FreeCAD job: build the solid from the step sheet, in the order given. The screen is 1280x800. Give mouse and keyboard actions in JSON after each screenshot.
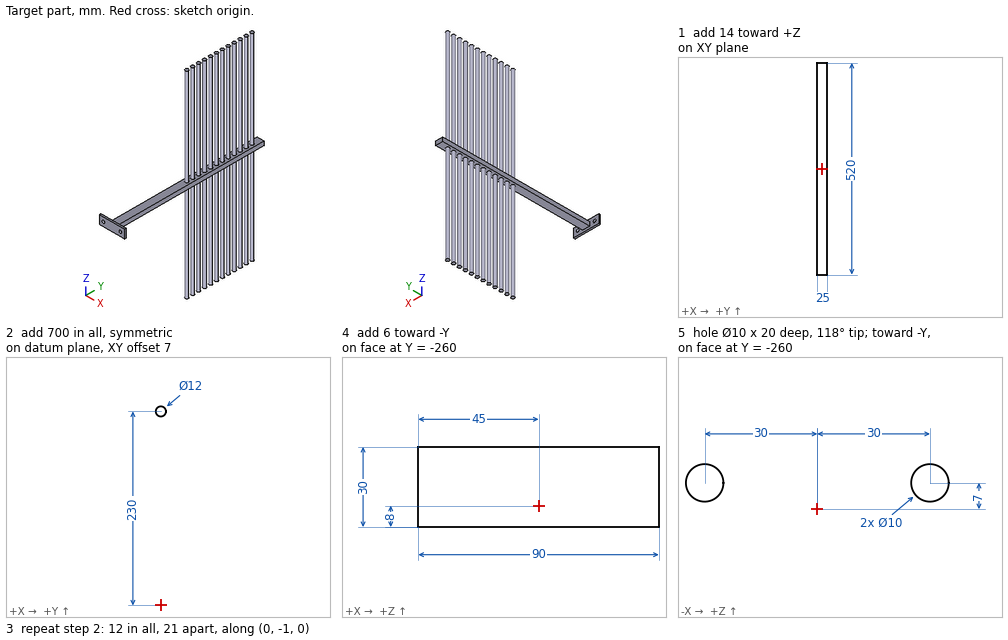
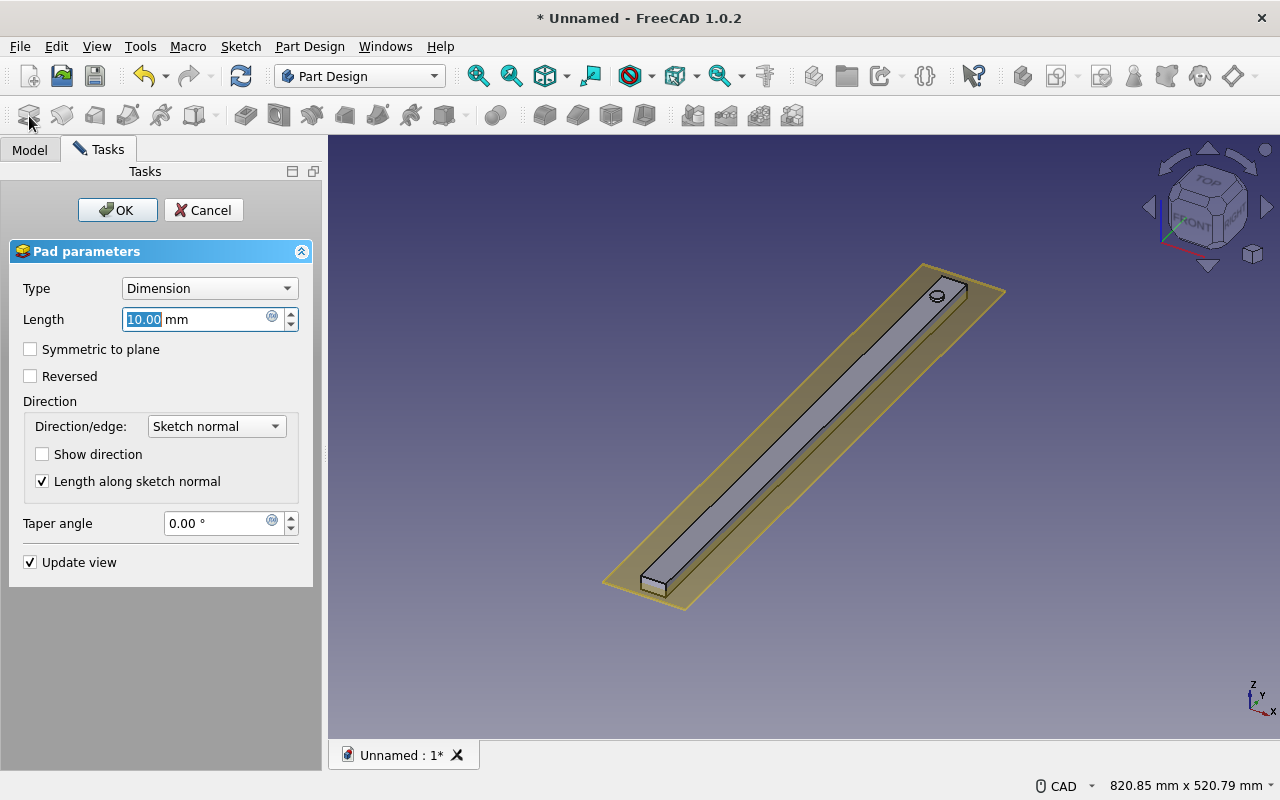
{"action": "type", "text": "700"}
{"action": "key", "text": "Tab"}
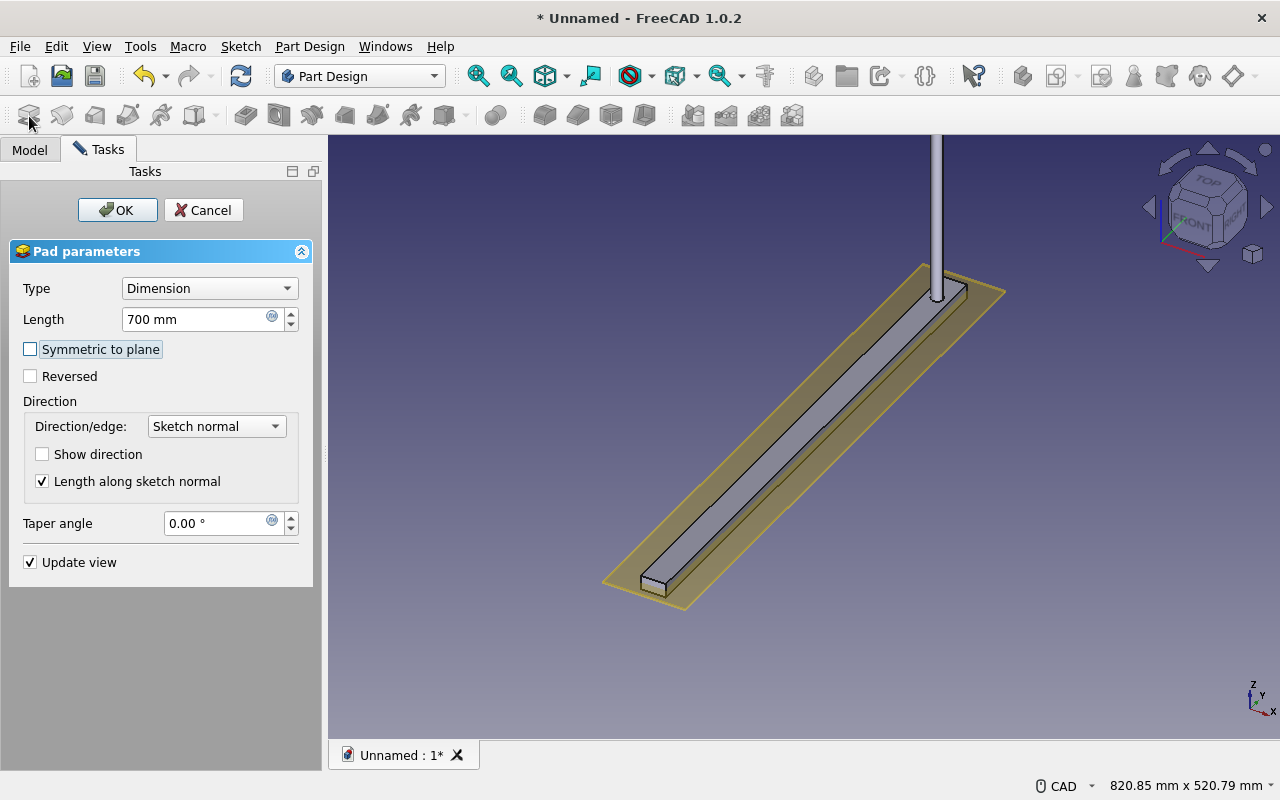
{"action": "left_click", "coordinate": [31, 349]}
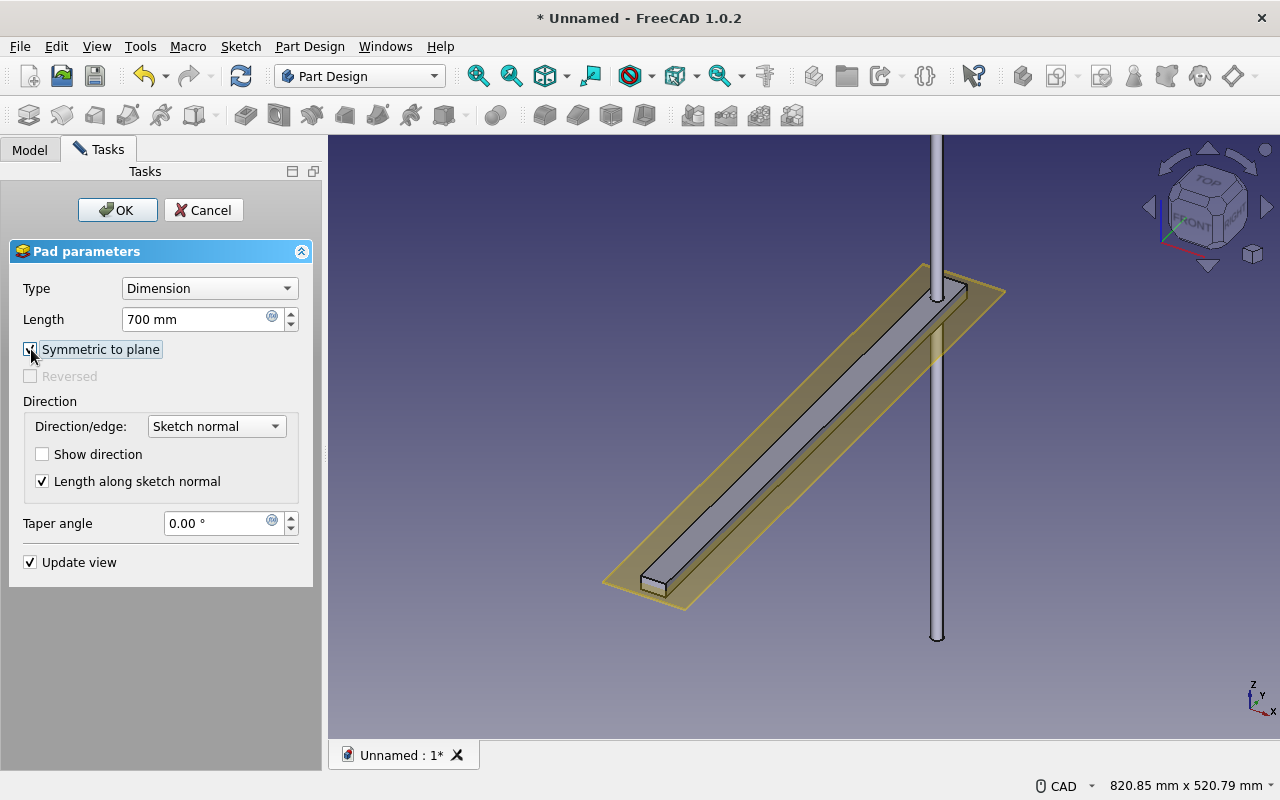
{"action": "left_click", "coordinate": [118, 210]}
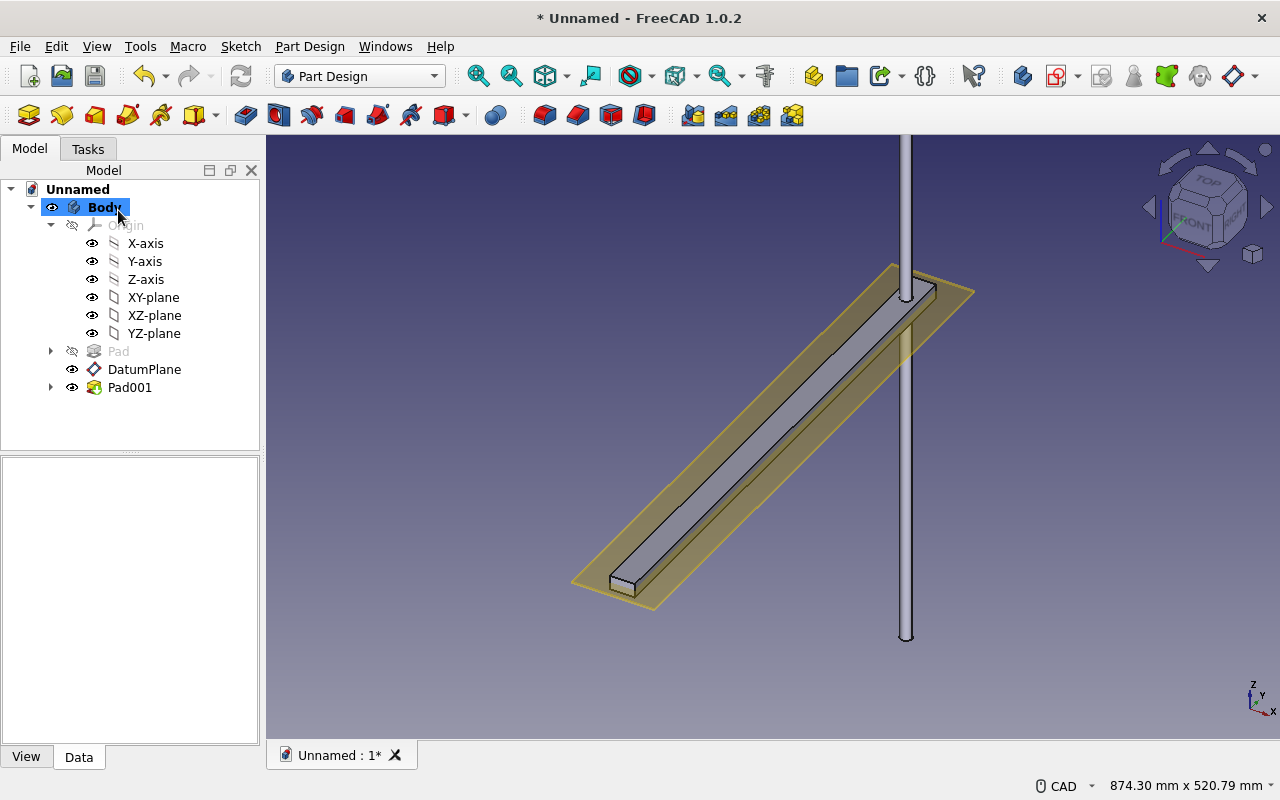
{"action": "left_click", "coordinate": [117, 369]}
{"action": "key", "text": "space"}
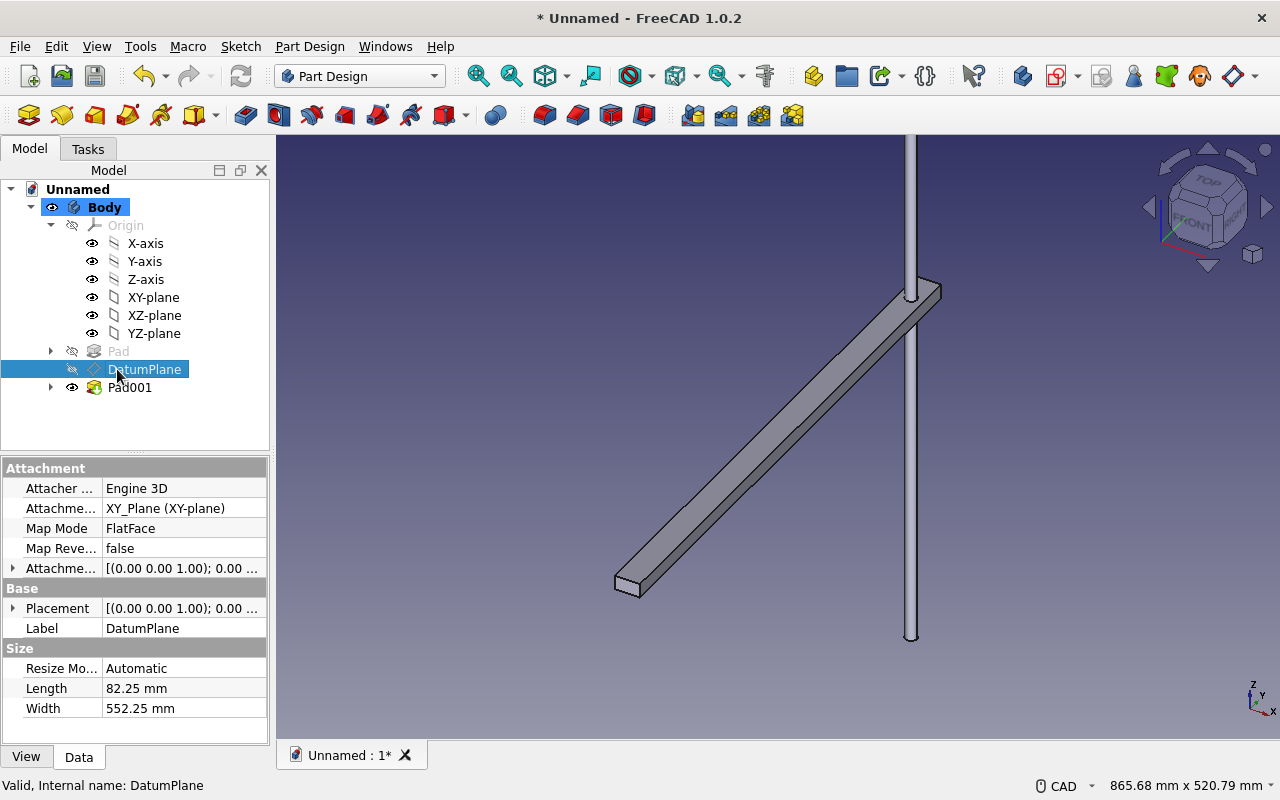
{"action": "left_click", "coordinate": [479, 76]}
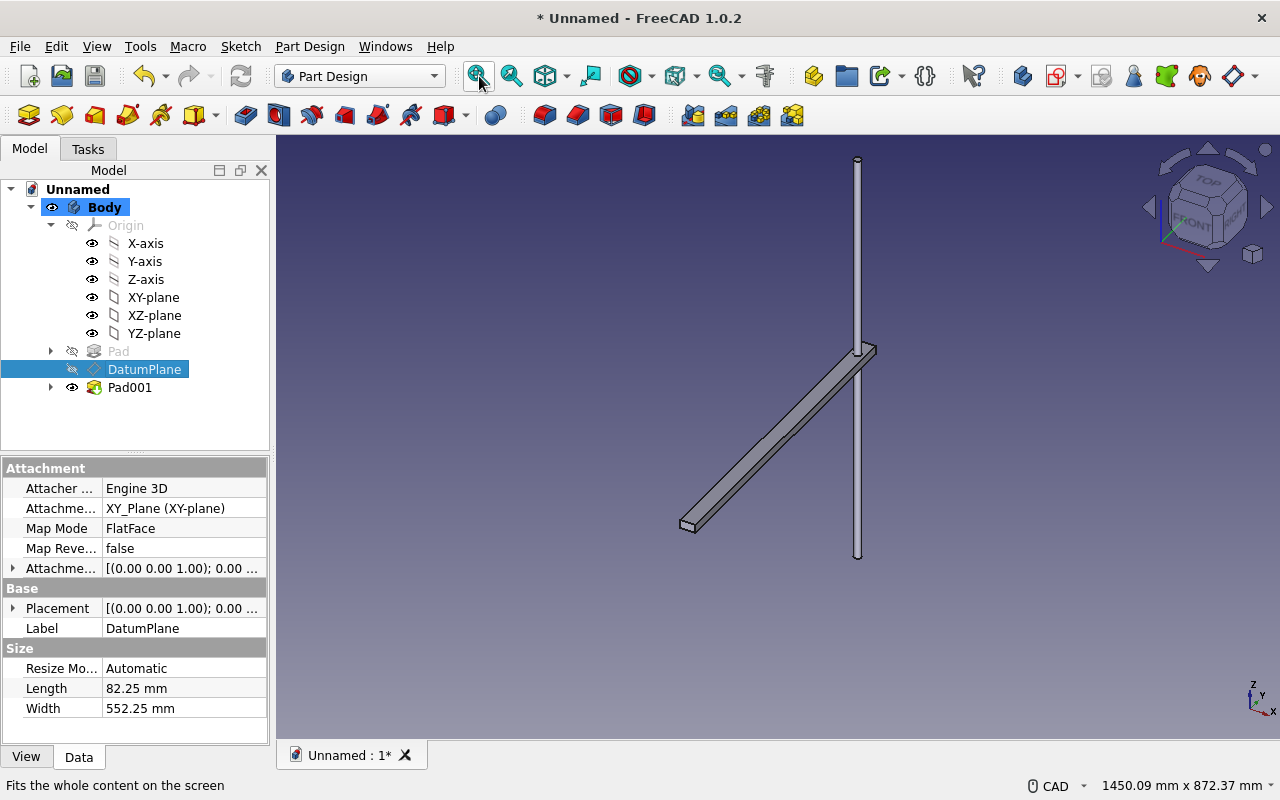
{"action": "left_click", "coordinate": [117, 387]}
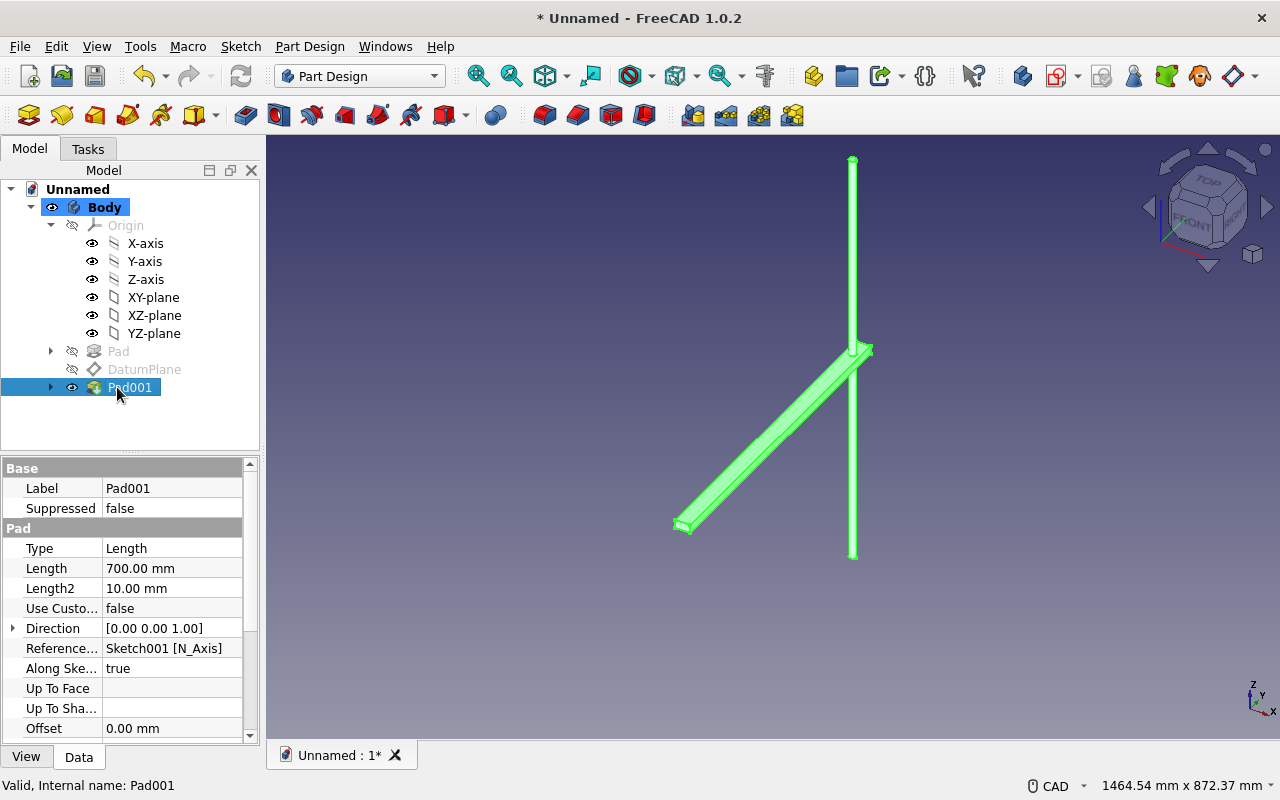
{"action": "left_click", "coordinate": [726, 116]}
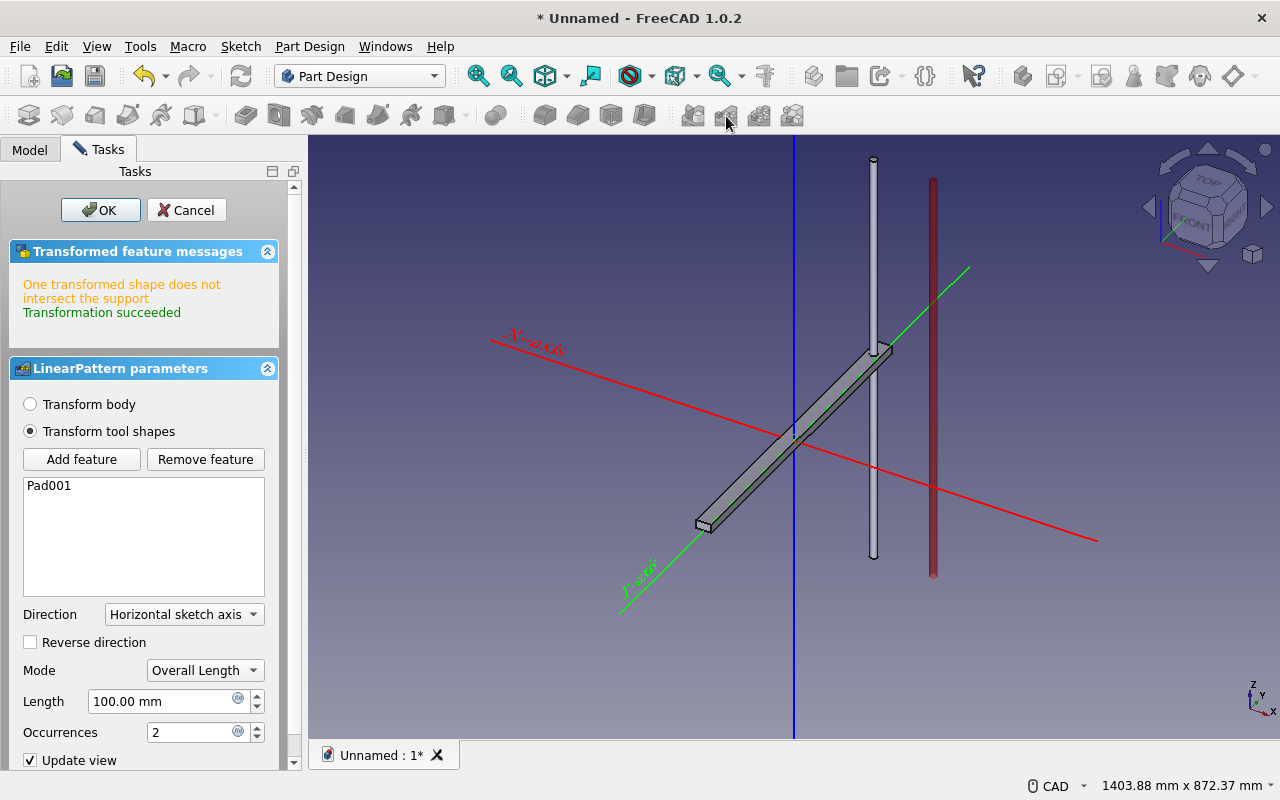
{"action": "left_click", "coordinate": [185, 614]}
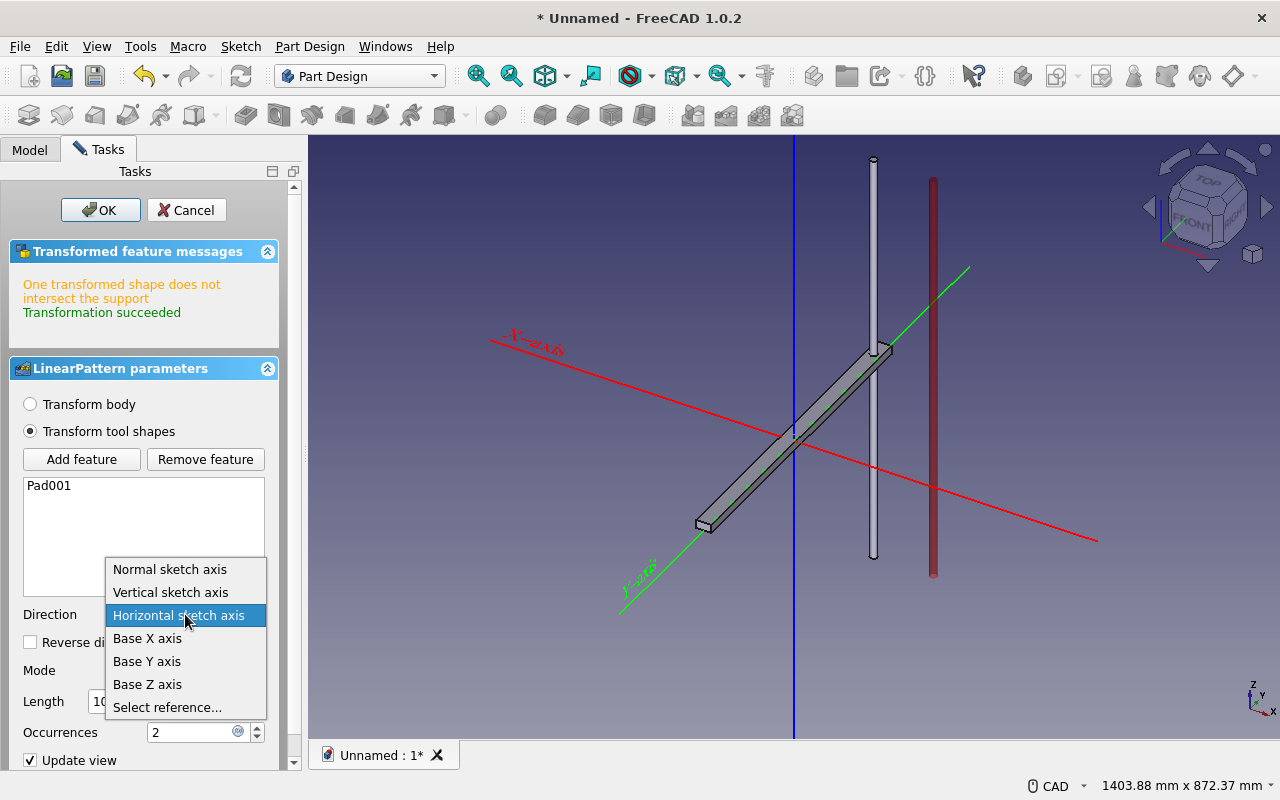
{"action": "left_click", "coordinate": [184, 662]}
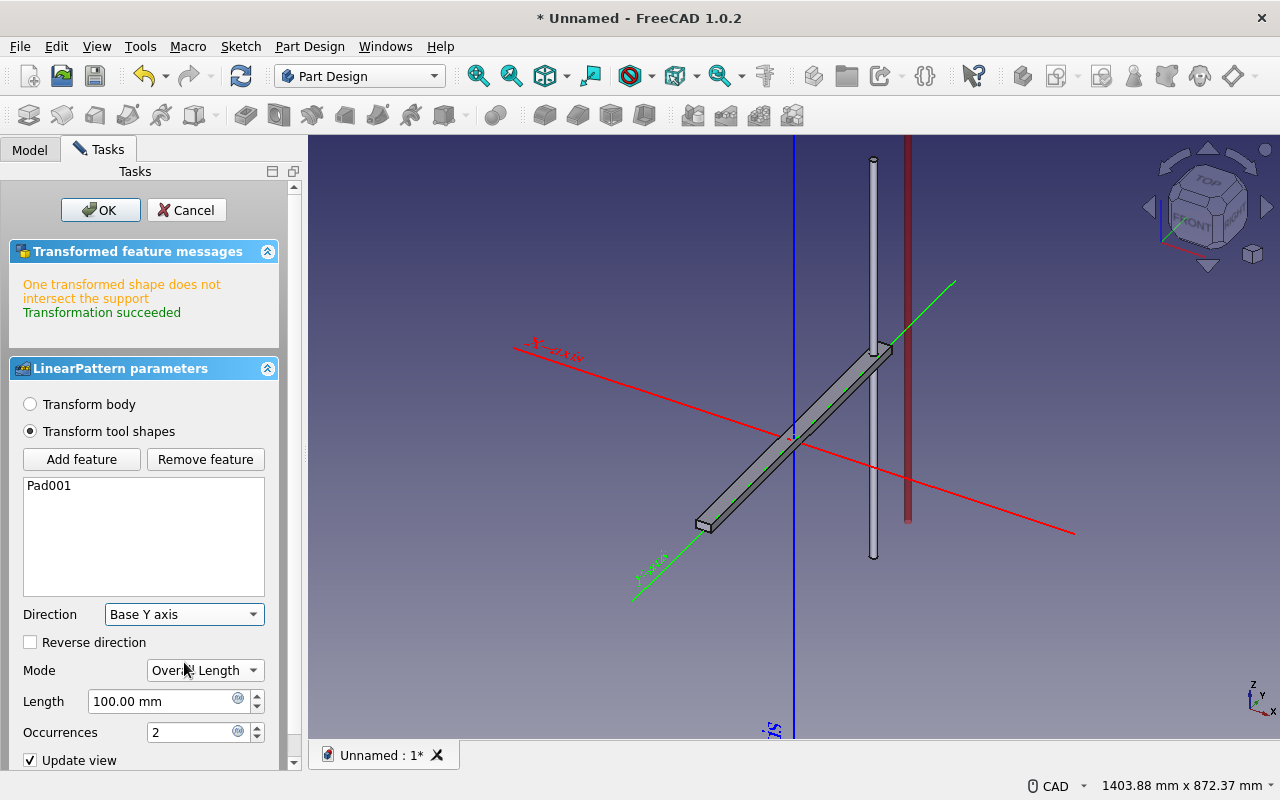
{"action": "left_click", "coordinate": [206, 670]}